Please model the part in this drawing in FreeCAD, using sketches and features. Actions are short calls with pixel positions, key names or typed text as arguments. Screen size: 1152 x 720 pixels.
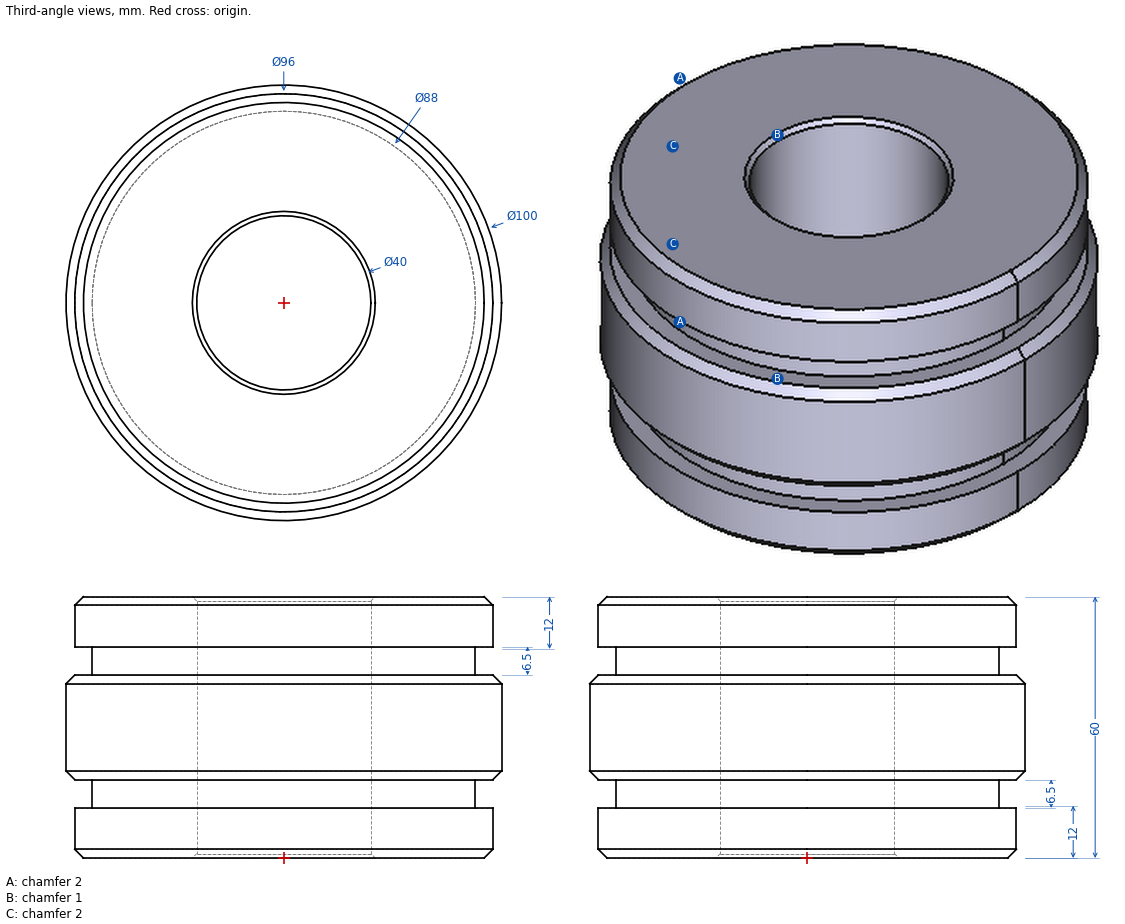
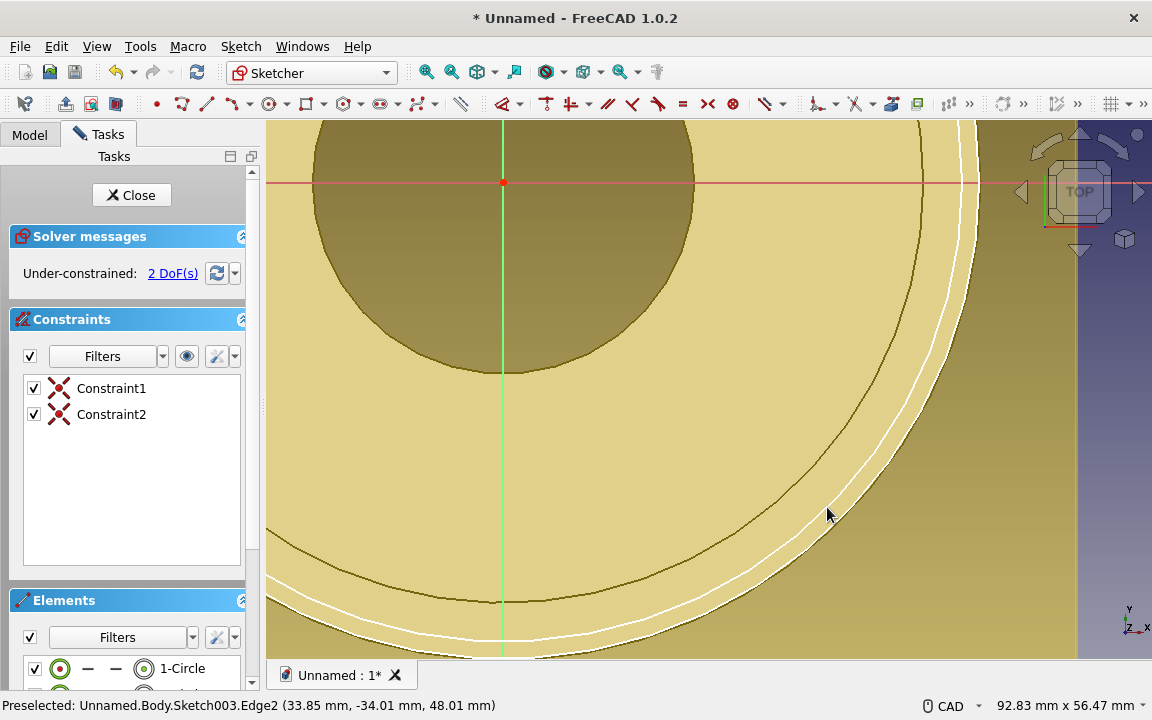
click(502, 104)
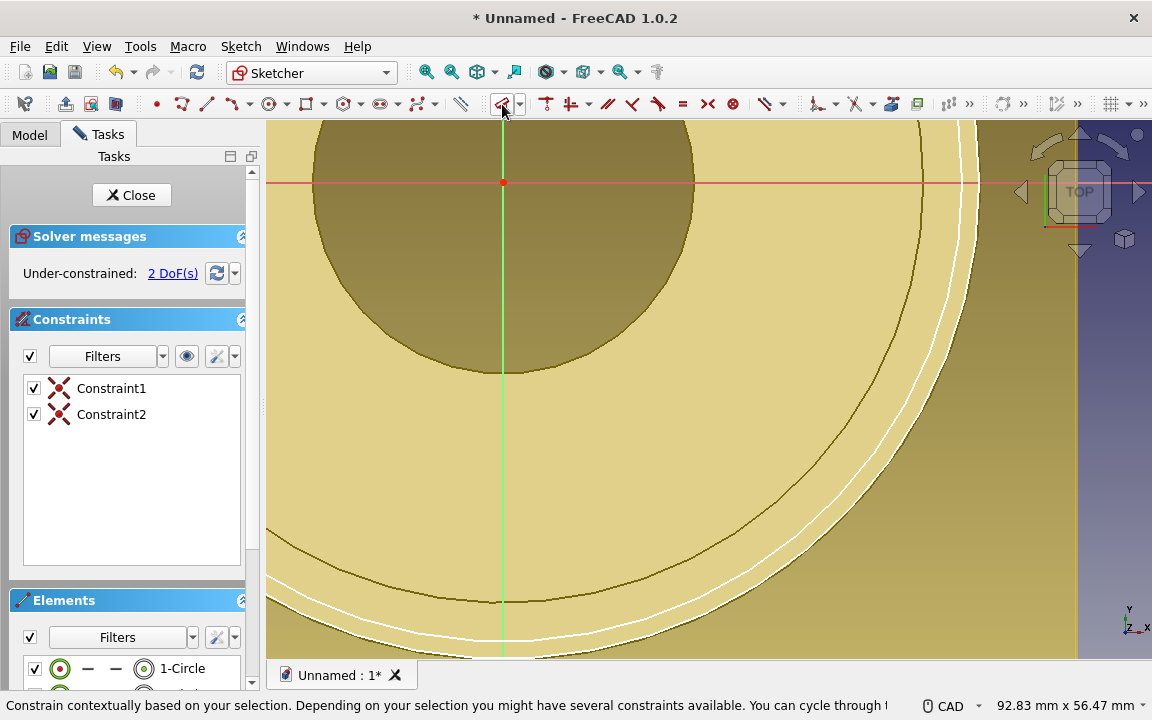
click(841, 518)
click(864, 541)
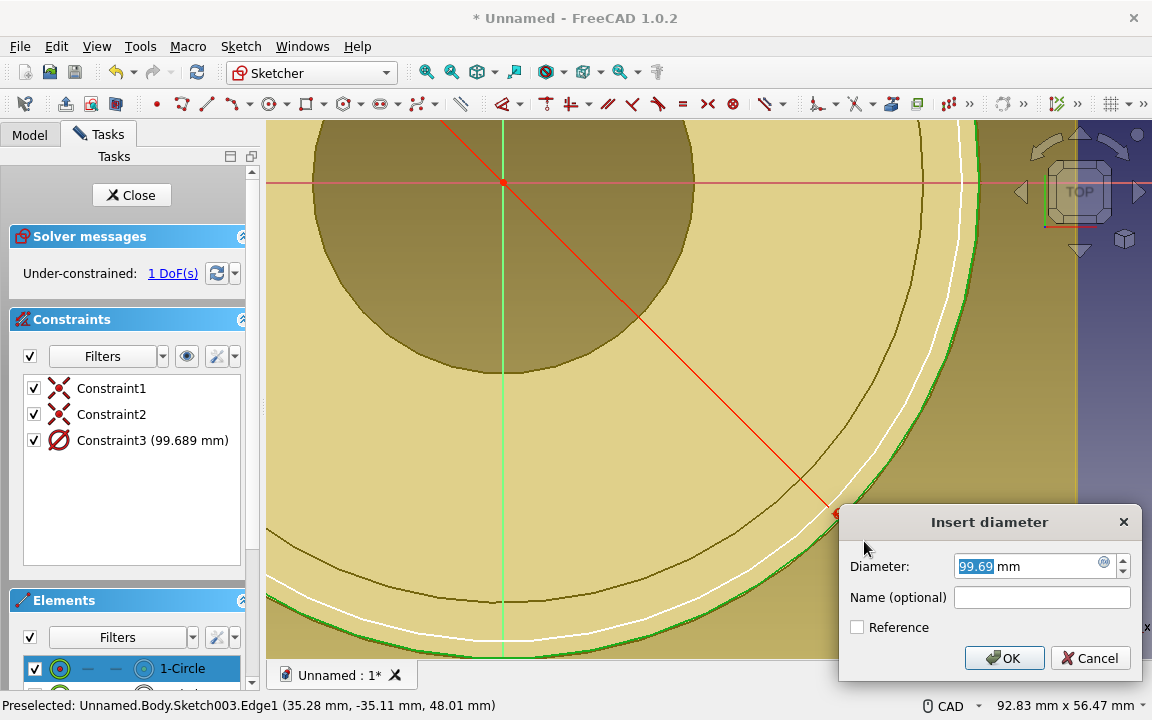
text(100)
key(Return)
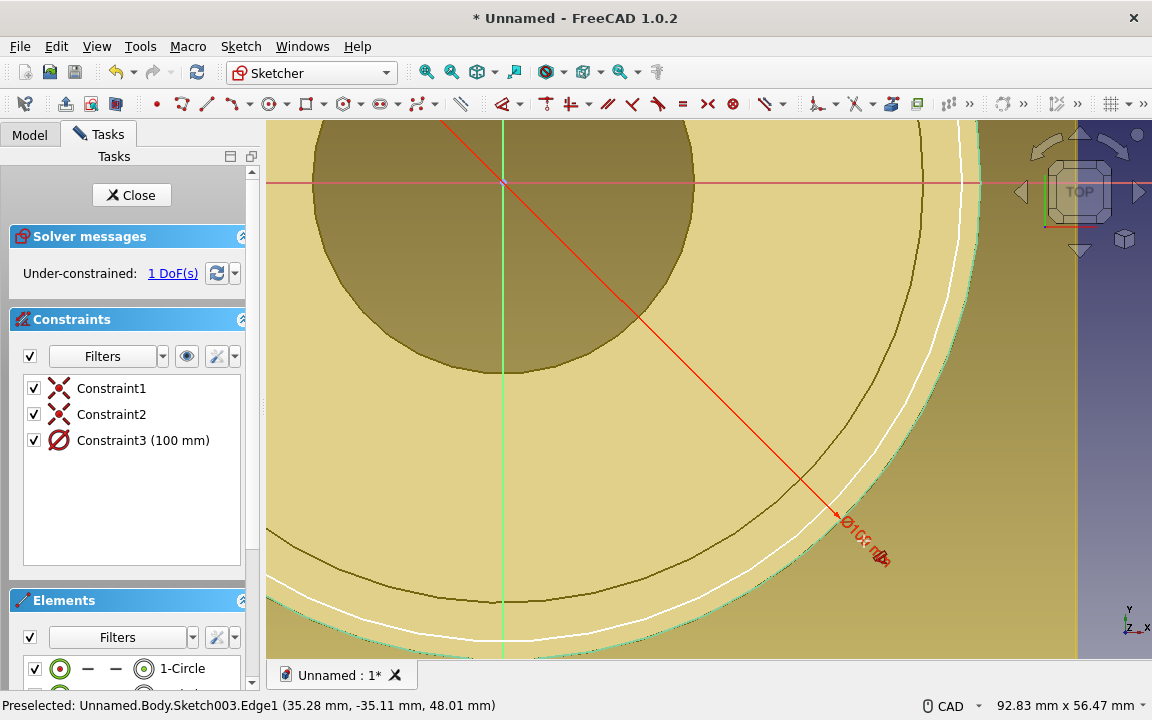
click(829, 506)
click(975, 319)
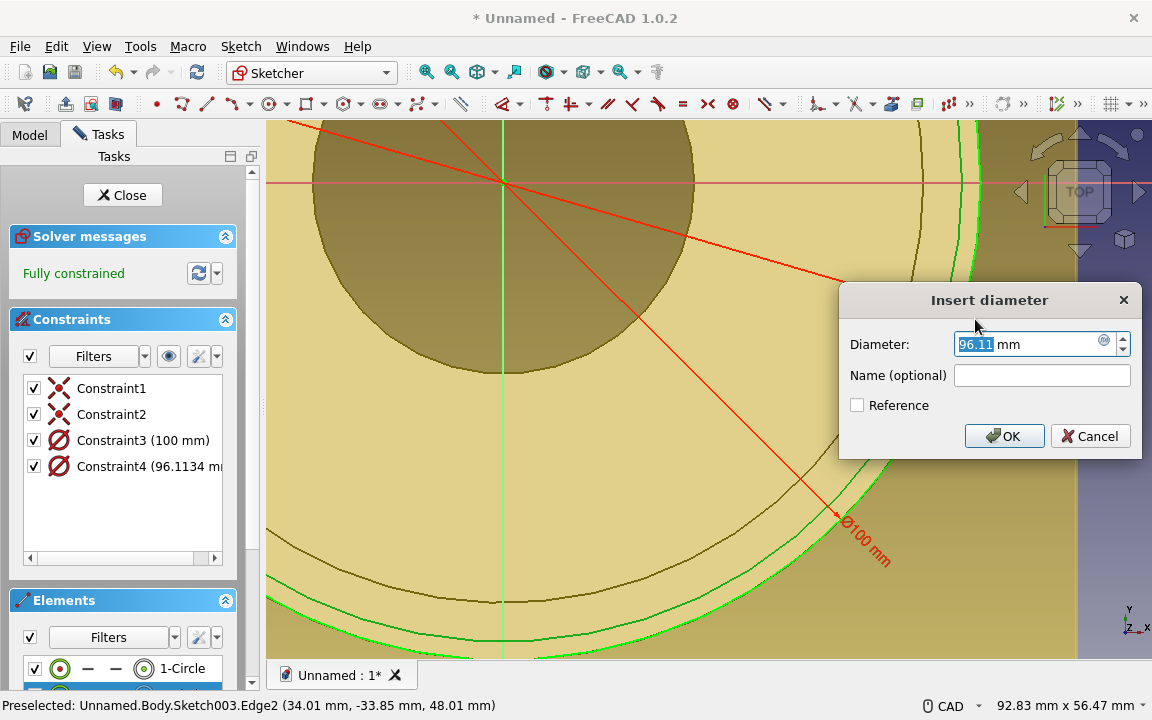
text(96)
key(Return)
key(Escape)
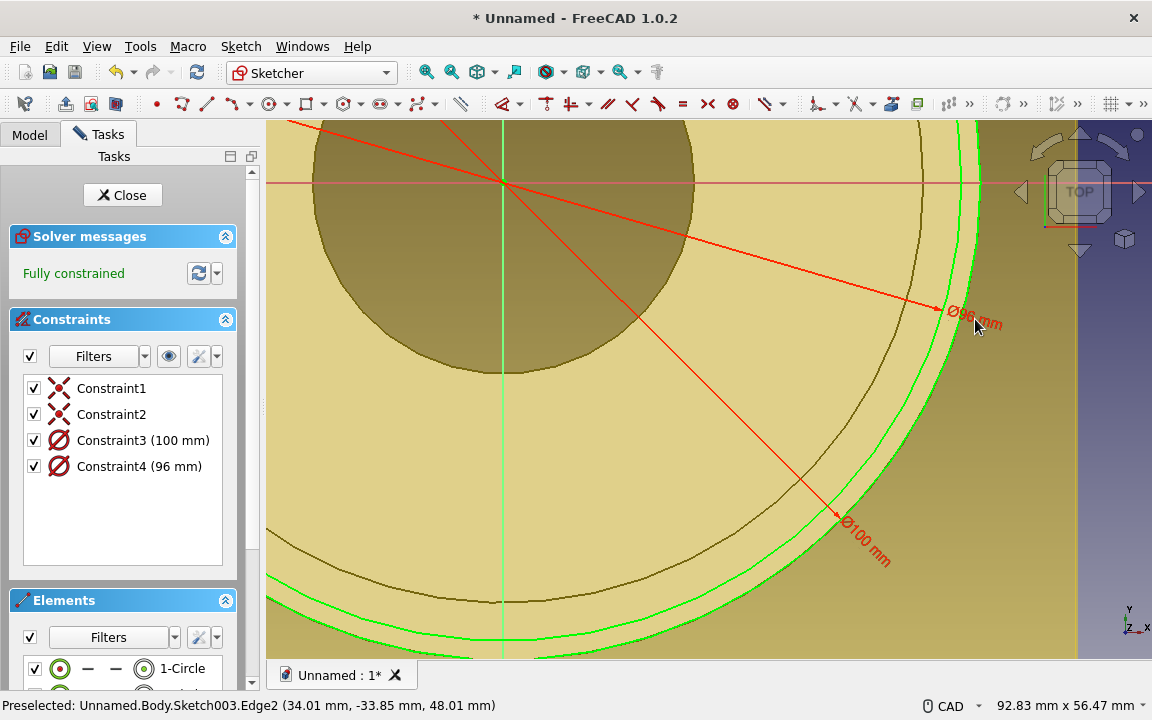
click(123, 195)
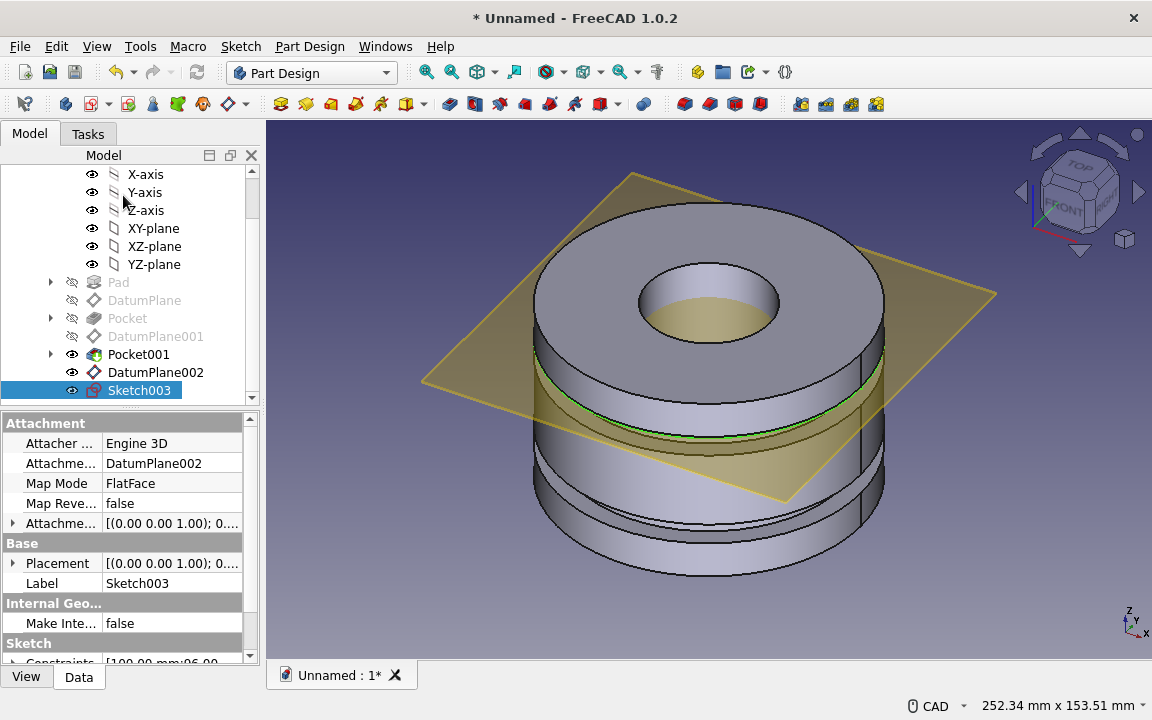
click(450, 104)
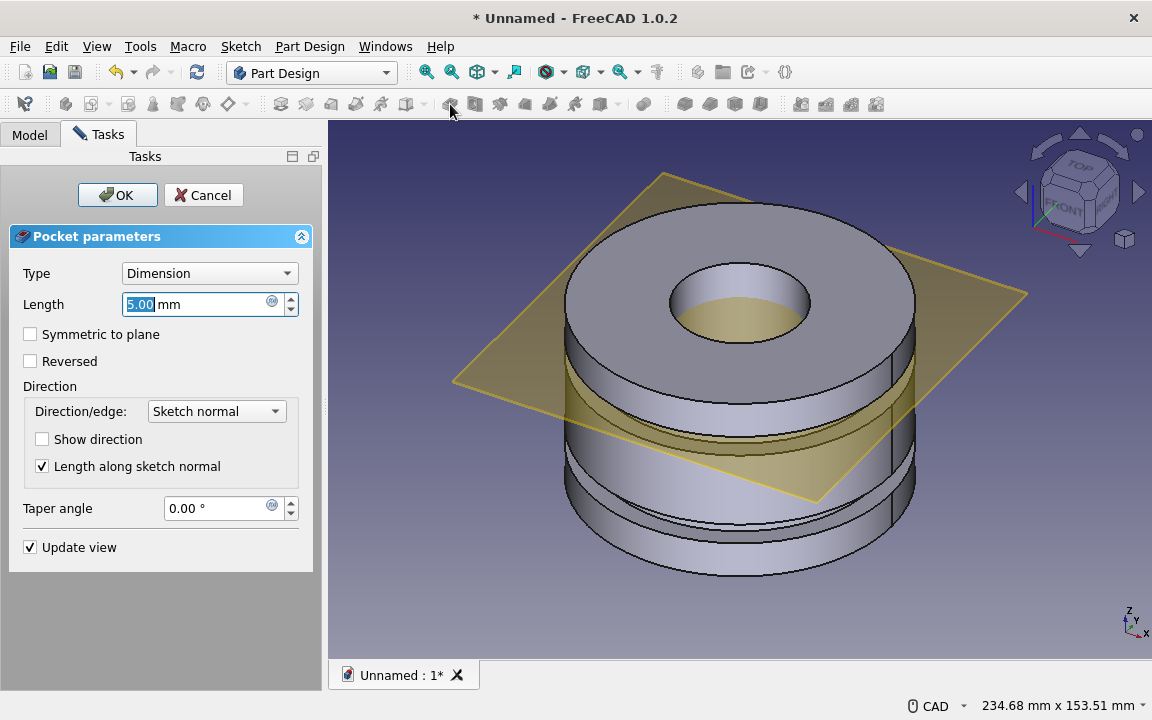
text(12)
key(Tab)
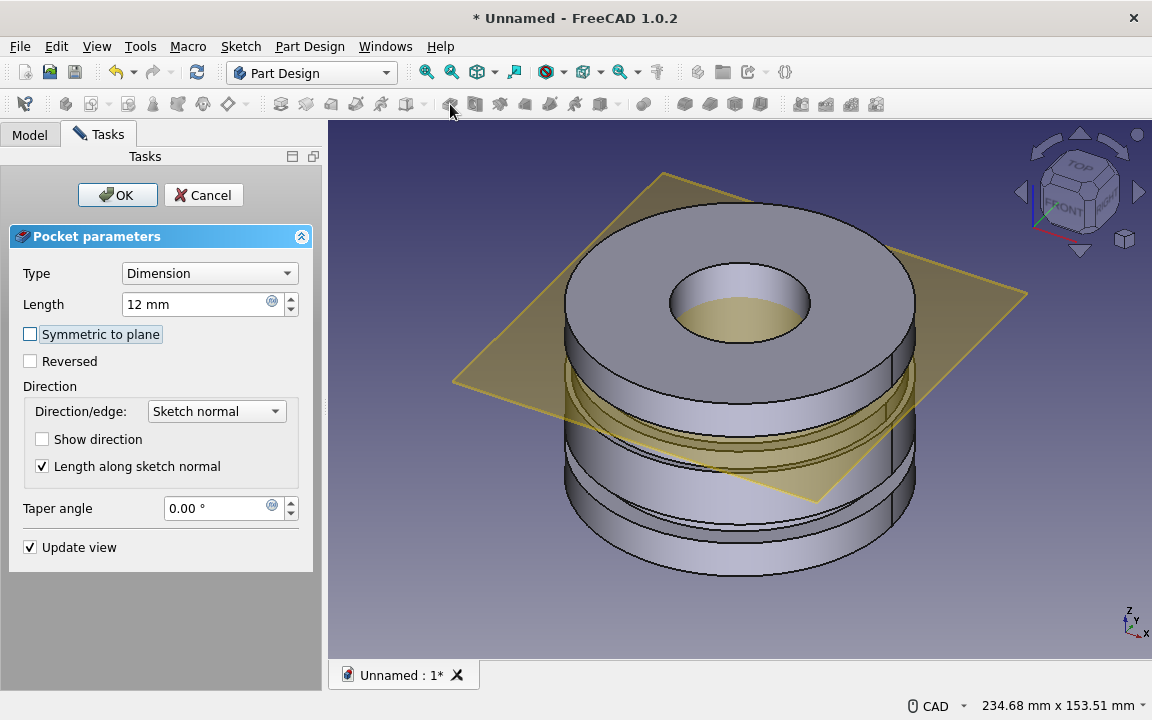
click(31, 361)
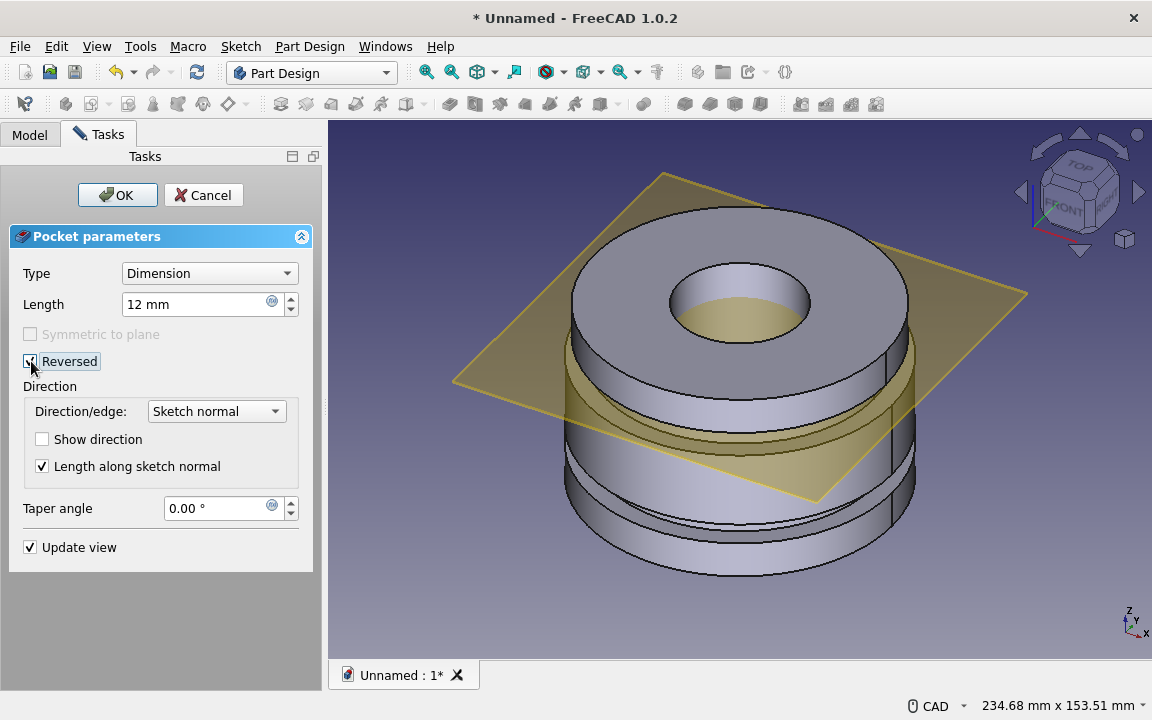
click(118, 195)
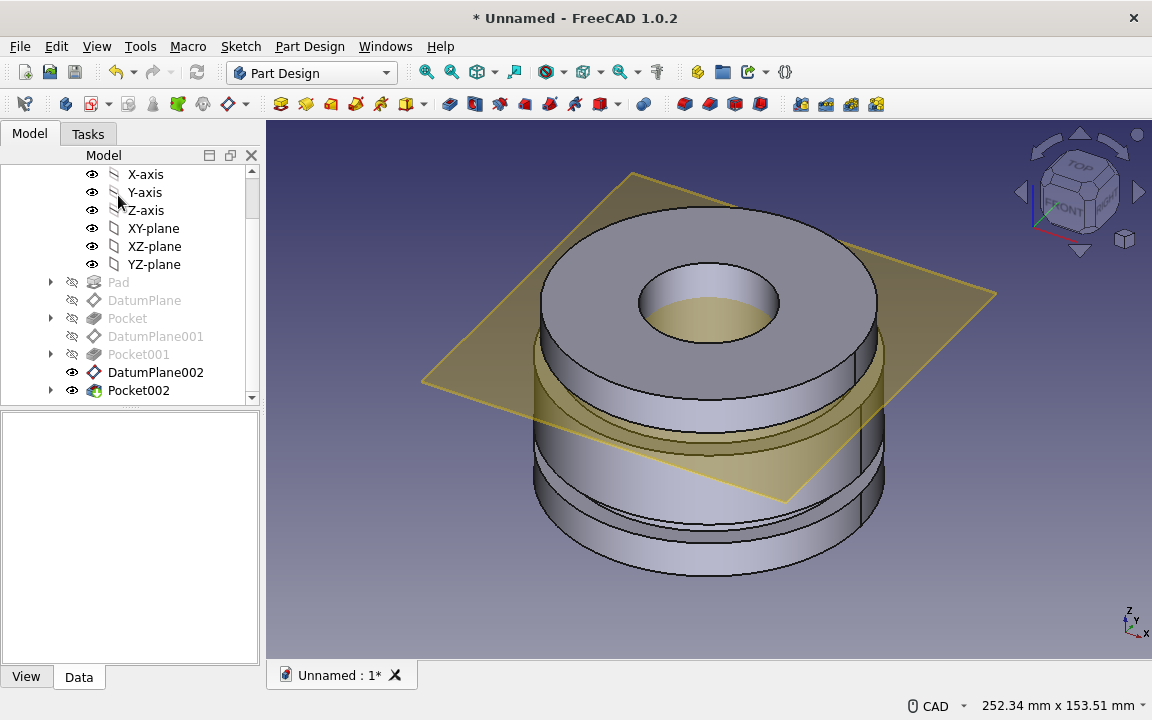
click(117, 372)
key(space)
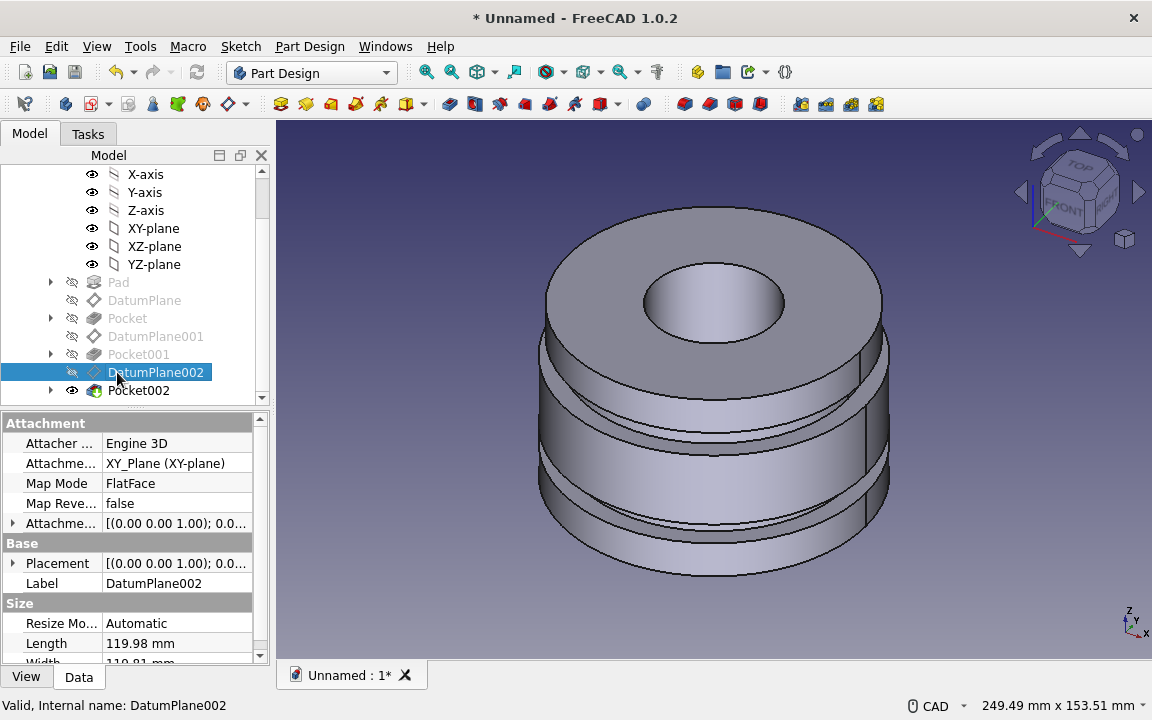
click(316, 619)